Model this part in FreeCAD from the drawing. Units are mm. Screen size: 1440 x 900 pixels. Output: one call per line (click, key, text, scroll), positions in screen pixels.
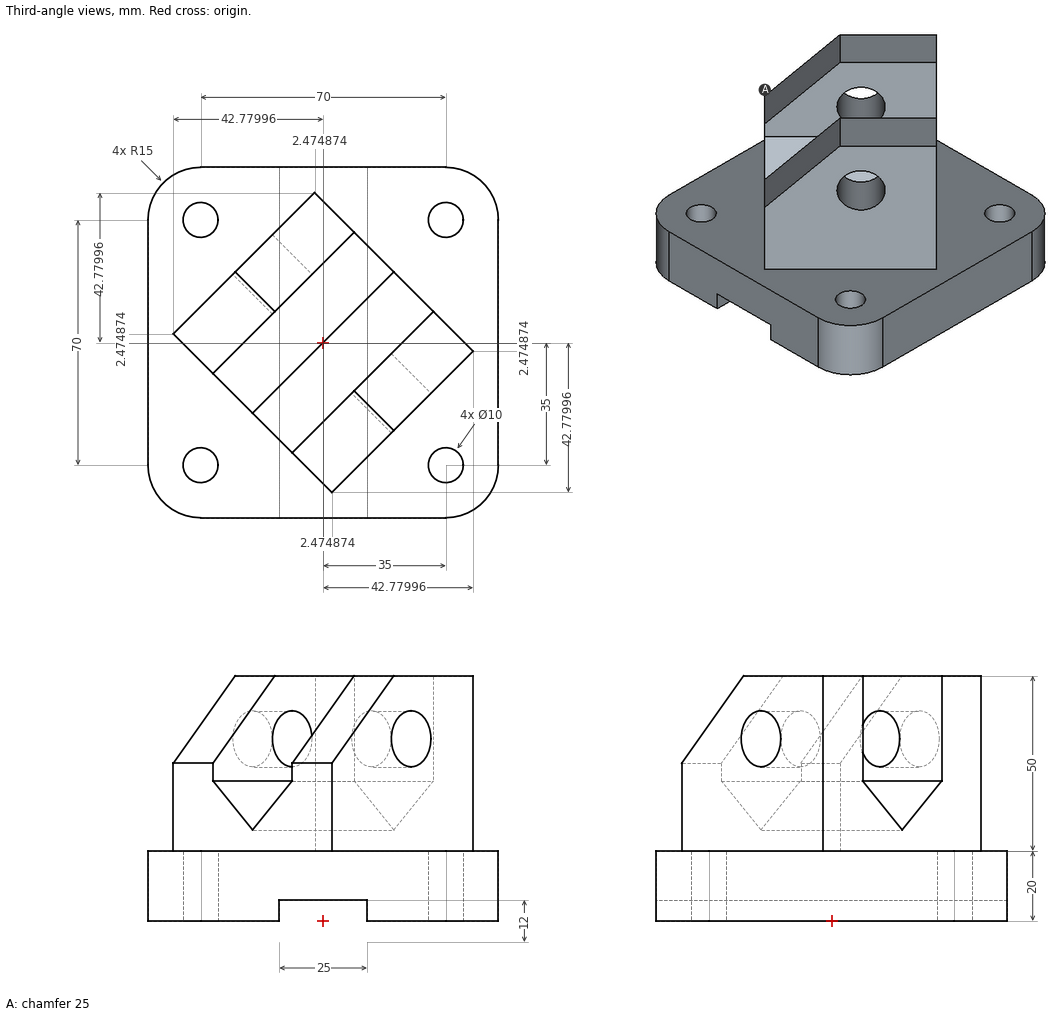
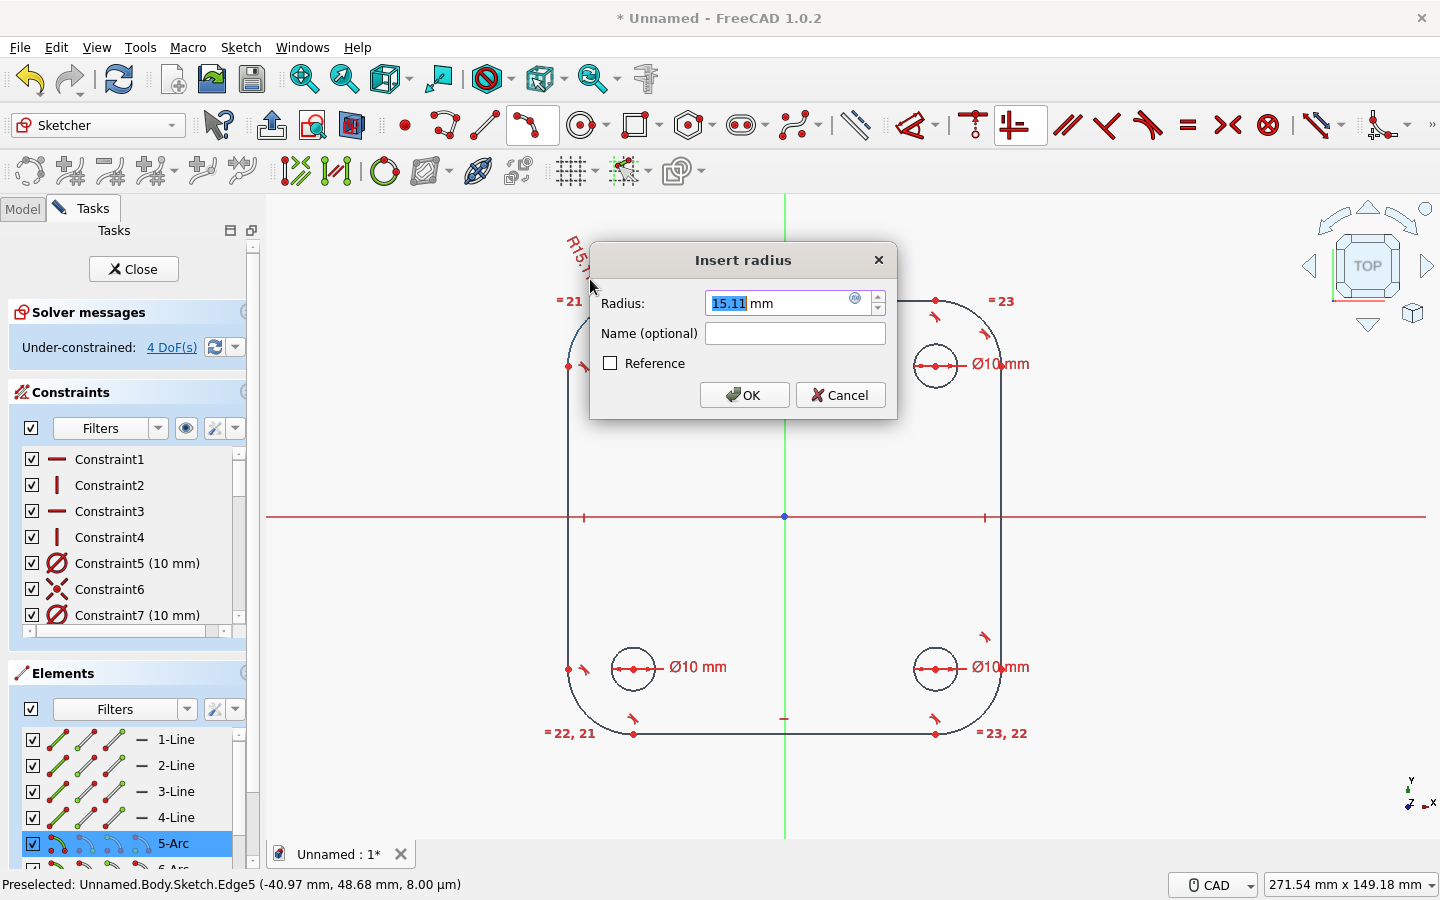
text(15)
key(Return)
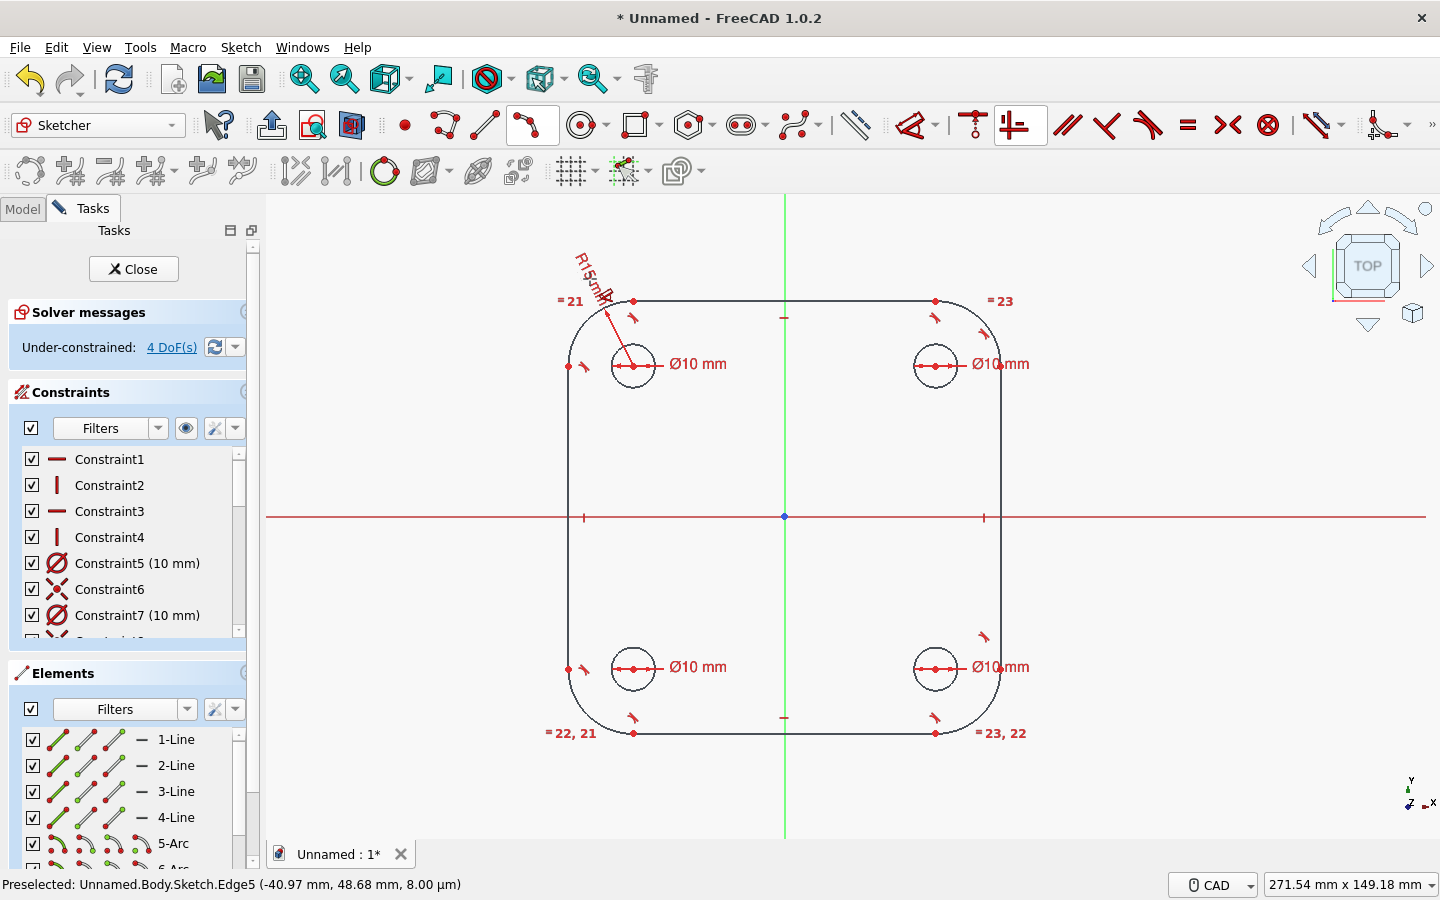
click(845, 301)
click(715, 267)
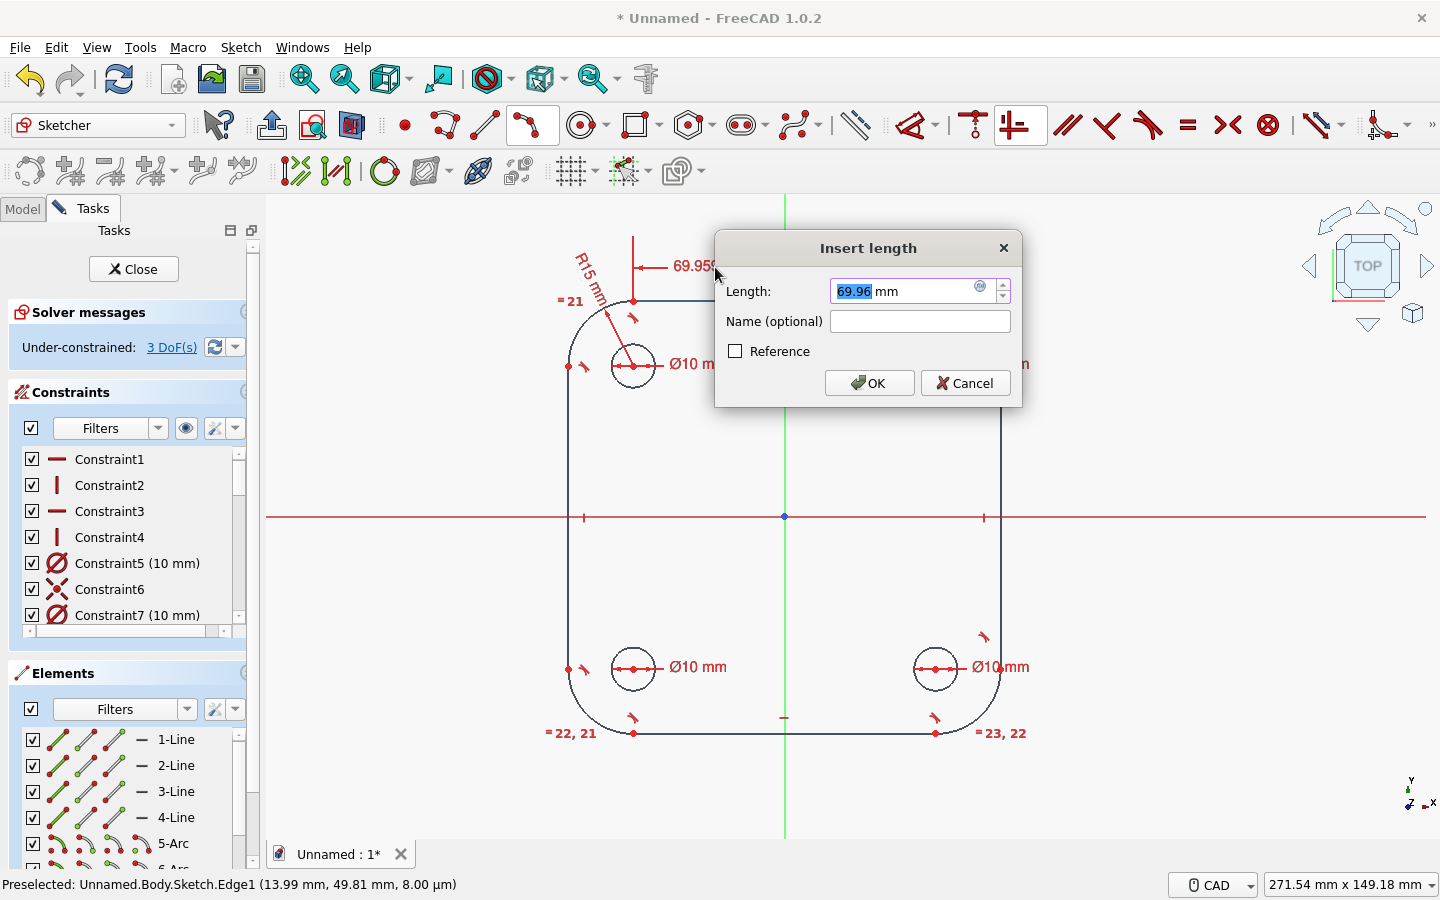
text(70)
key(Return)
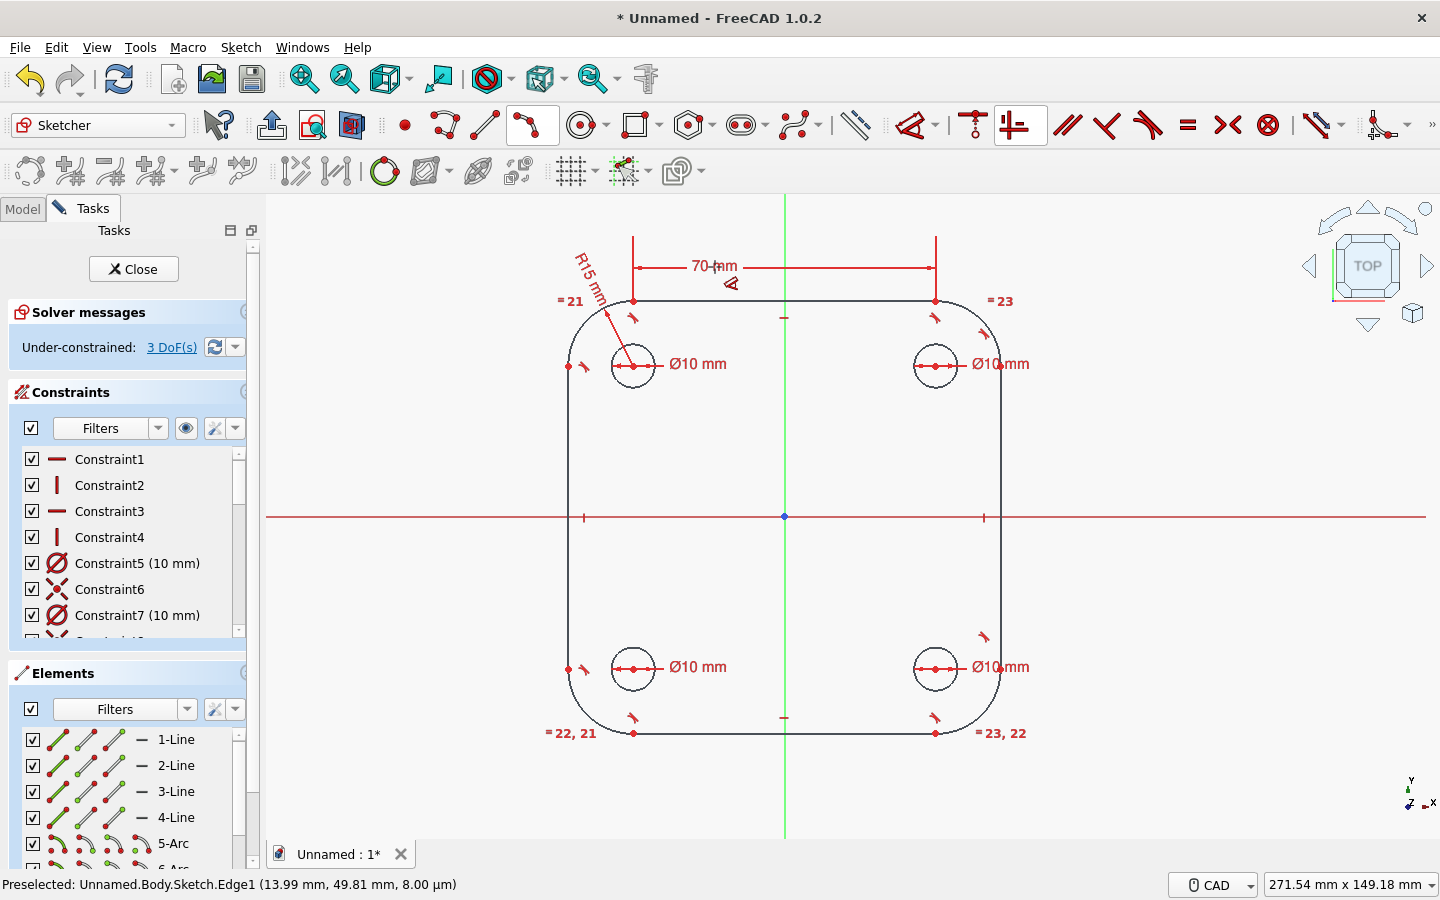
click(568, 457)
click(534, 448)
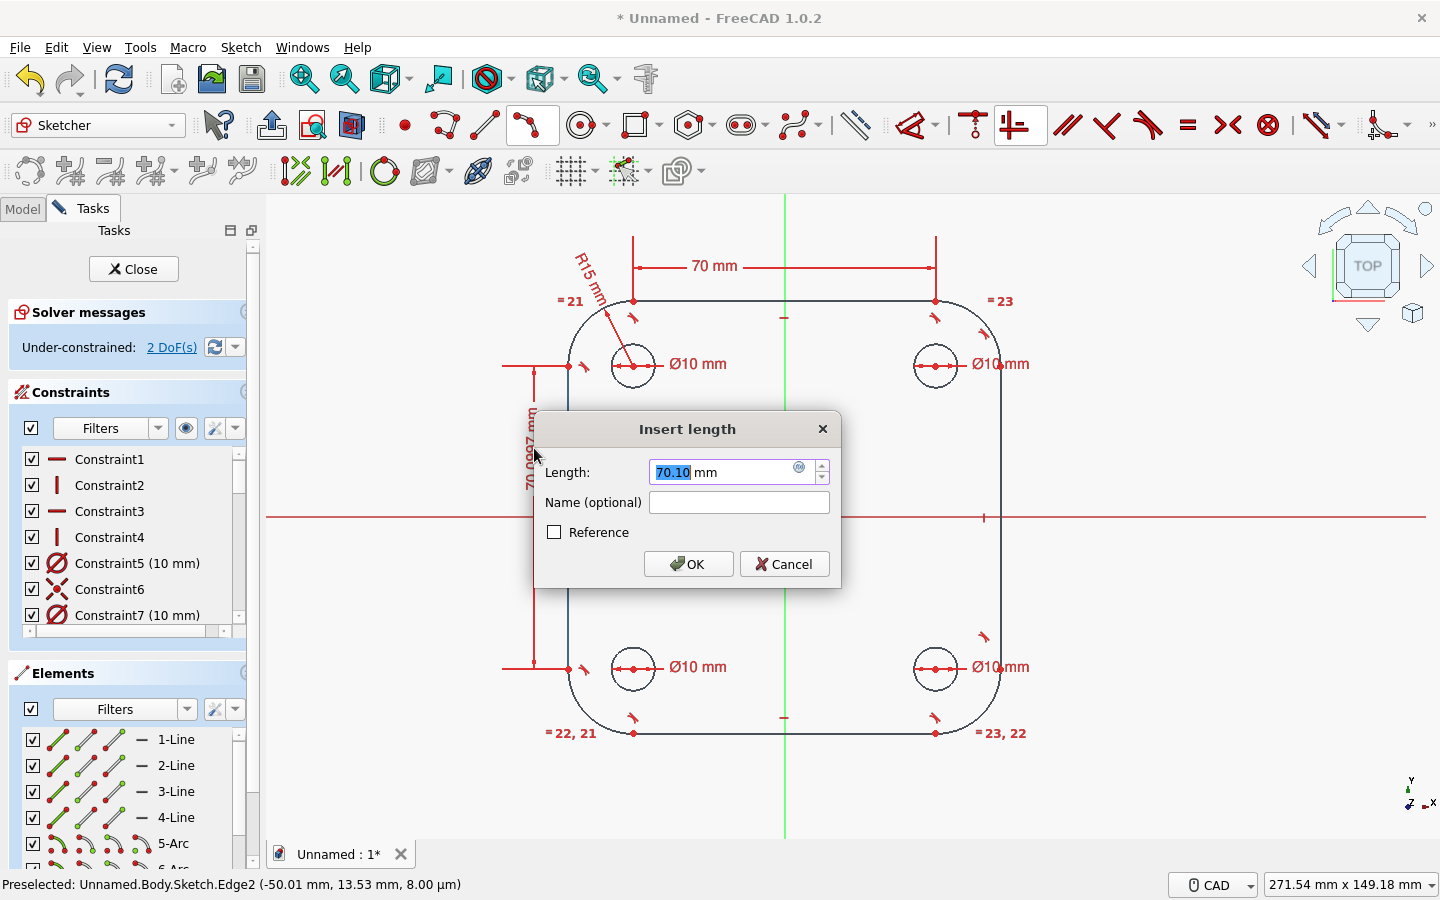
text(70)
key(Return)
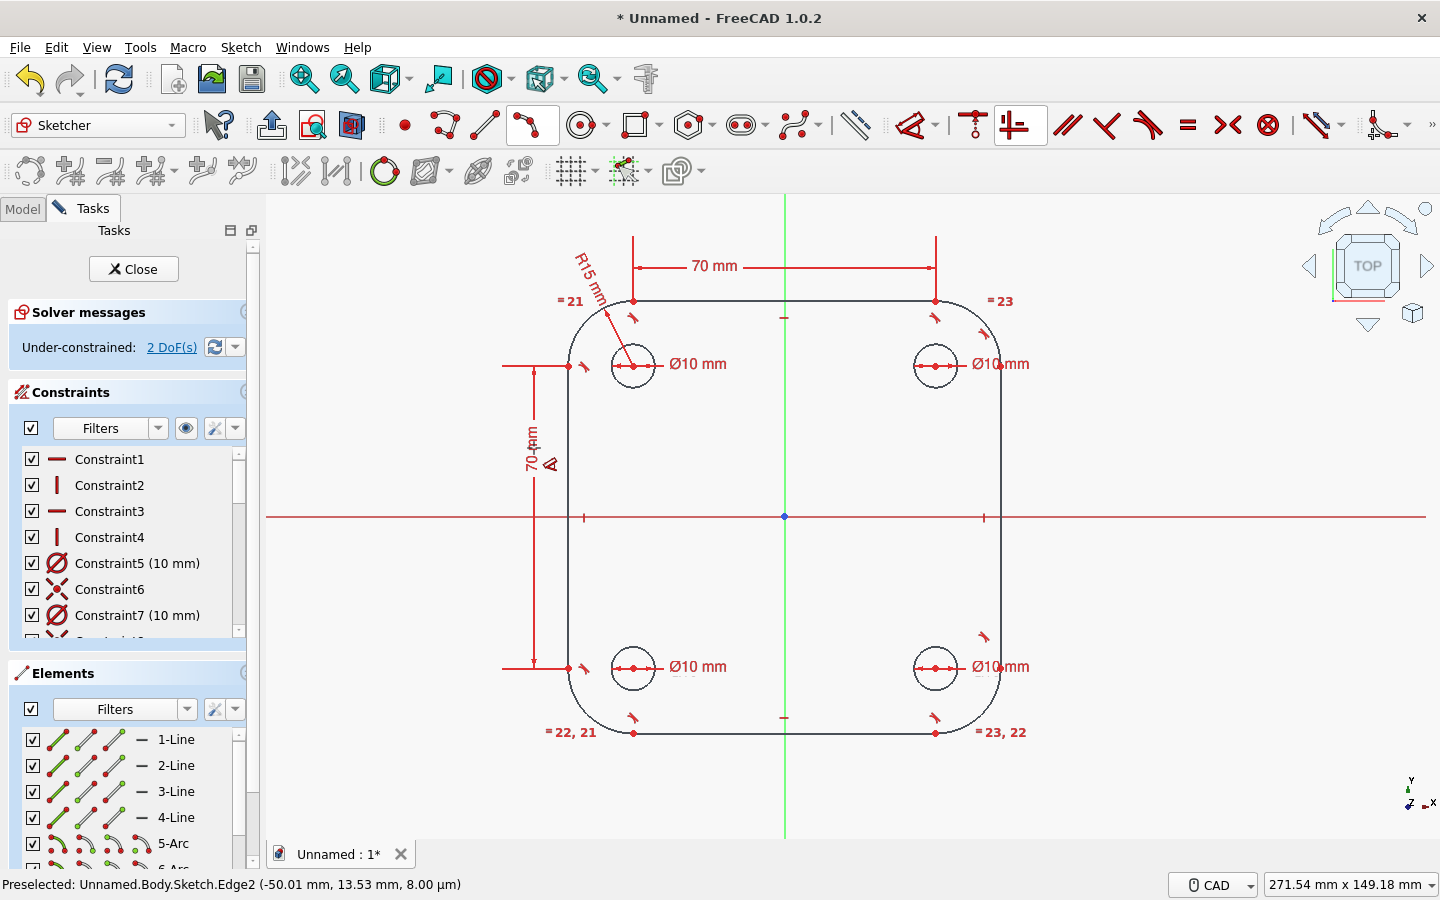
click(936, 669)
click(860, 703)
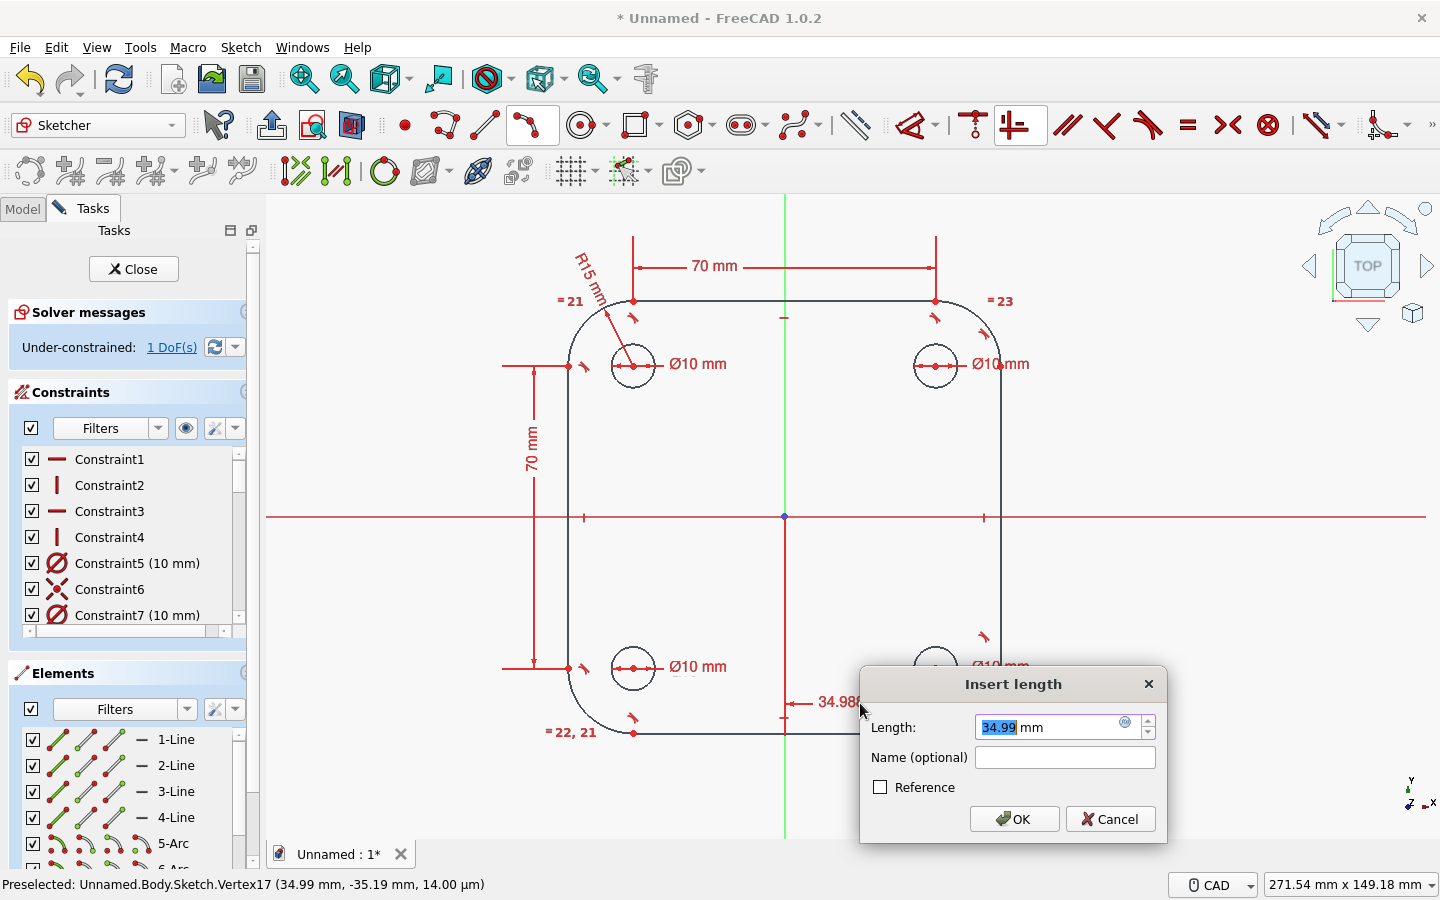
text(35)
key(Return)